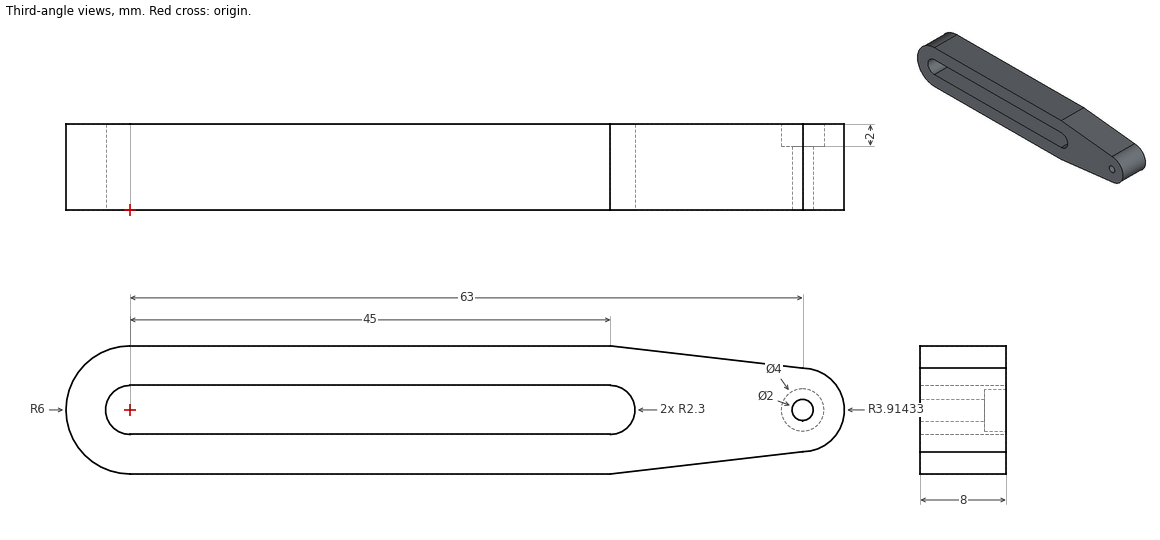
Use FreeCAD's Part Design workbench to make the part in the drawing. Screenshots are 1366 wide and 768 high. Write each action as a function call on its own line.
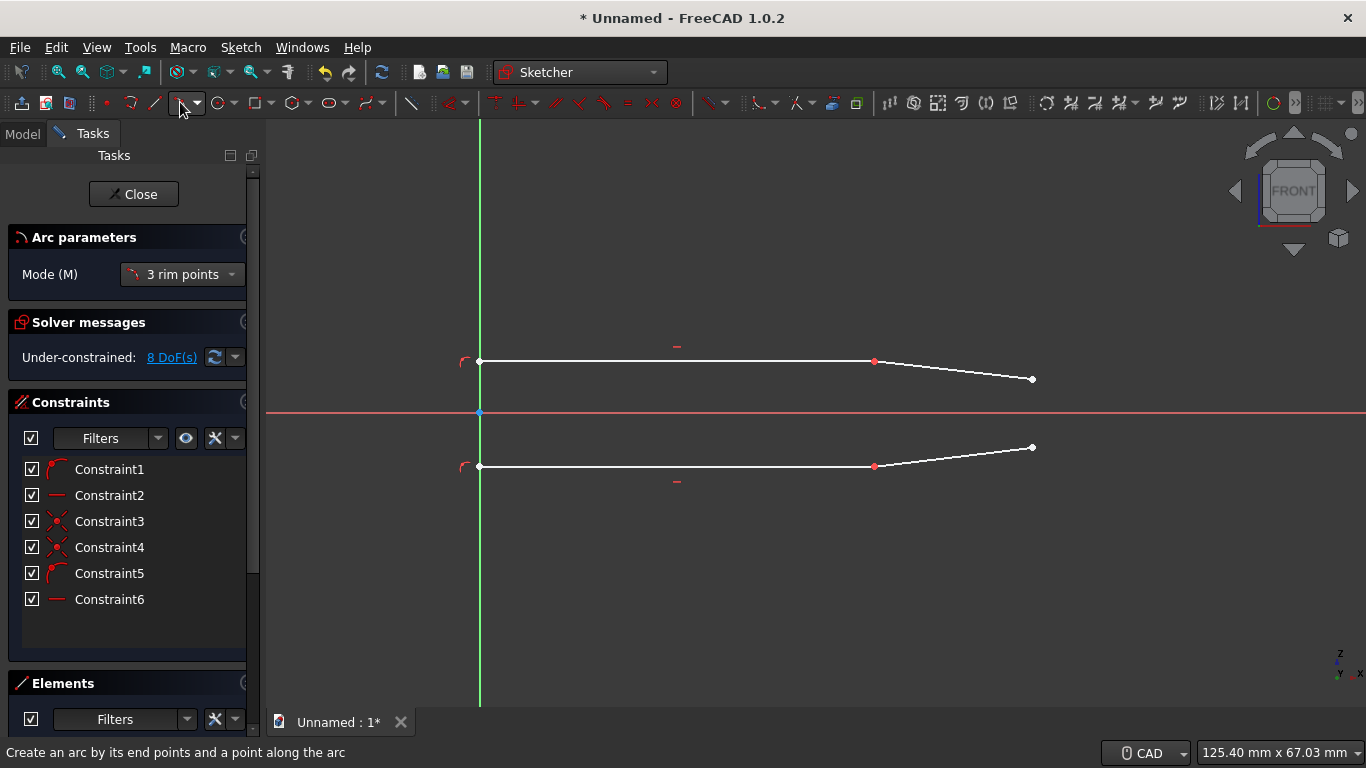
click(1032, 379)
click(1032, 448)
click(1060, 433)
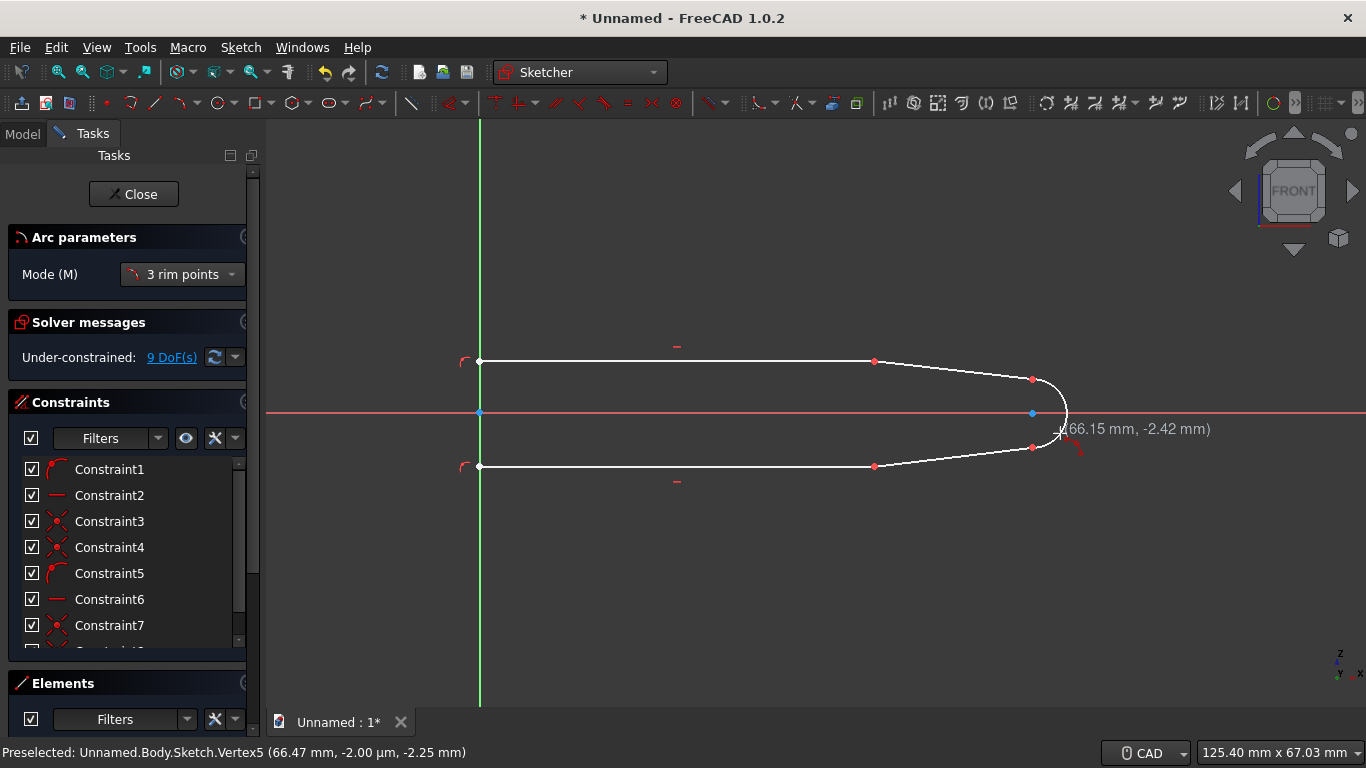
click(480, 467)
click(480, 361)
click(430, 396)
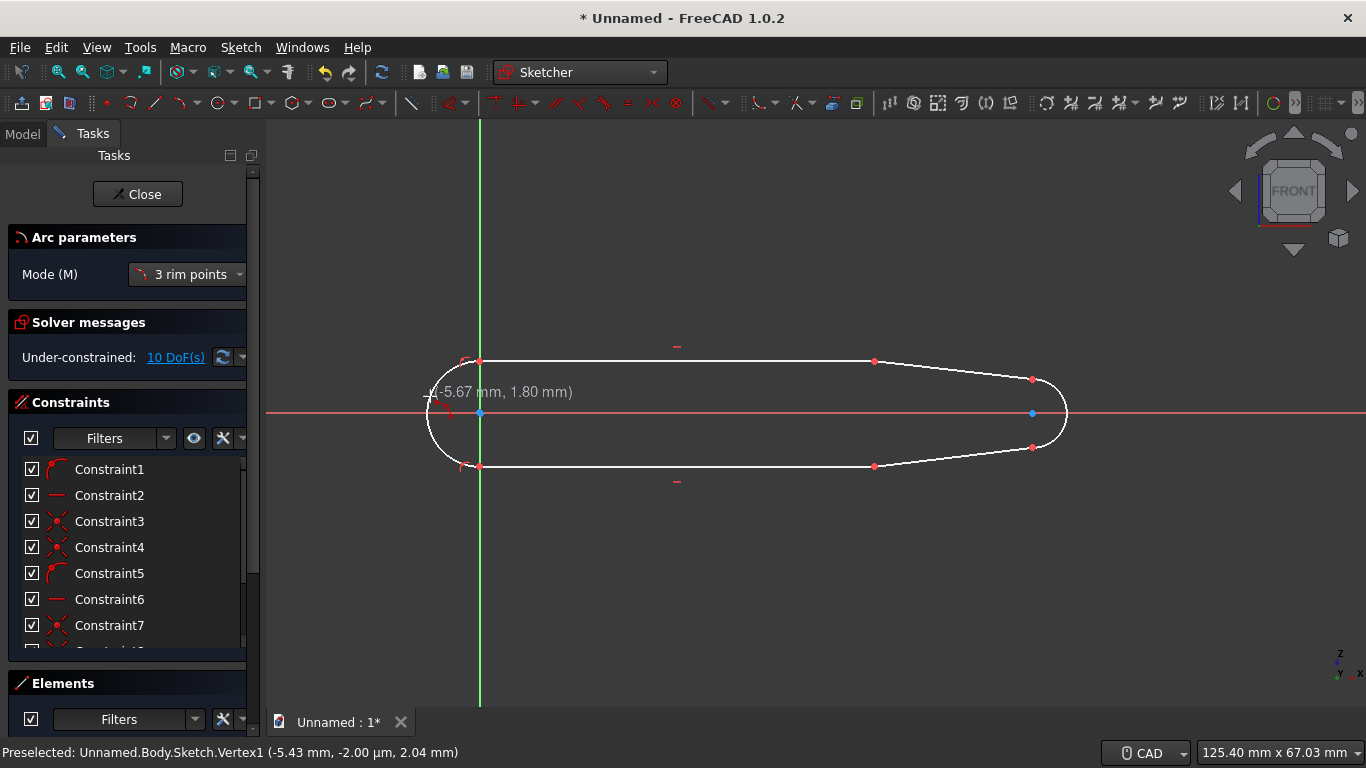
click(330, 104)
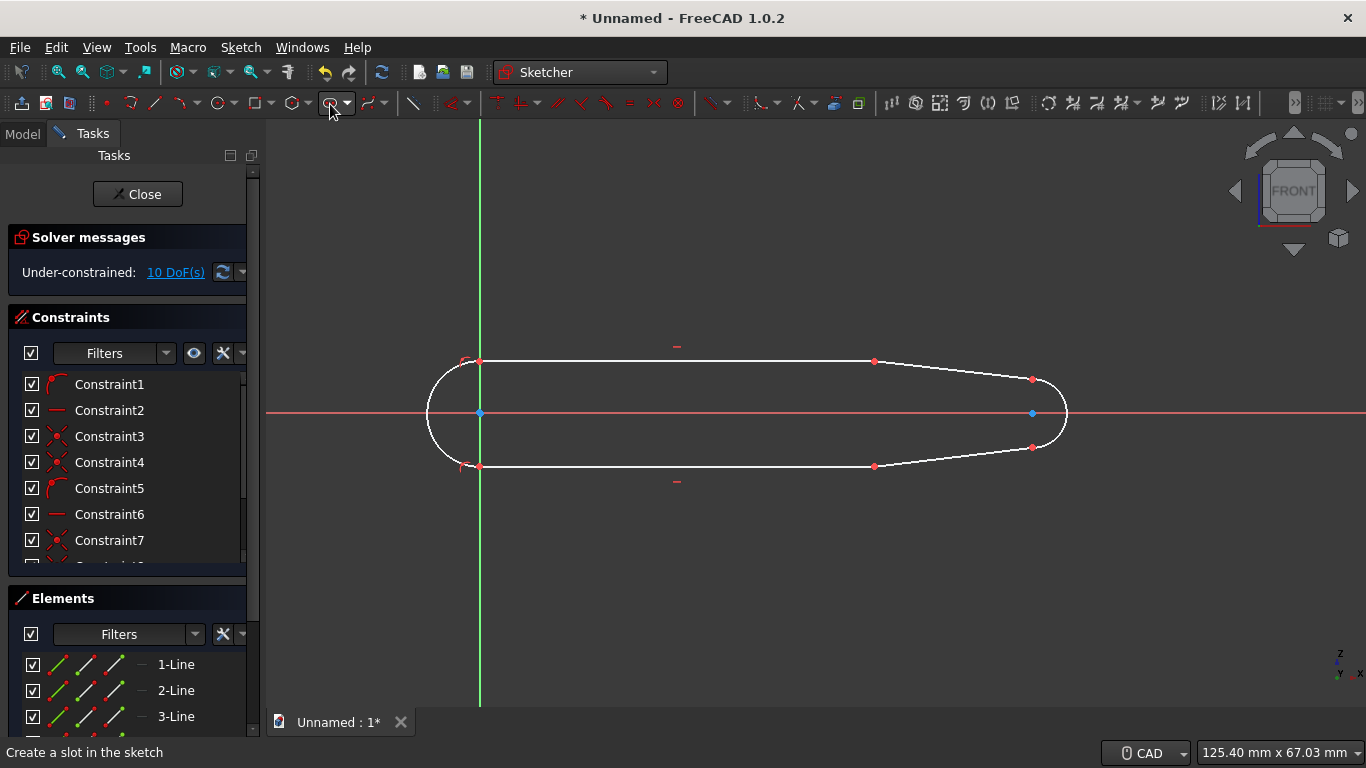
click(480, 413)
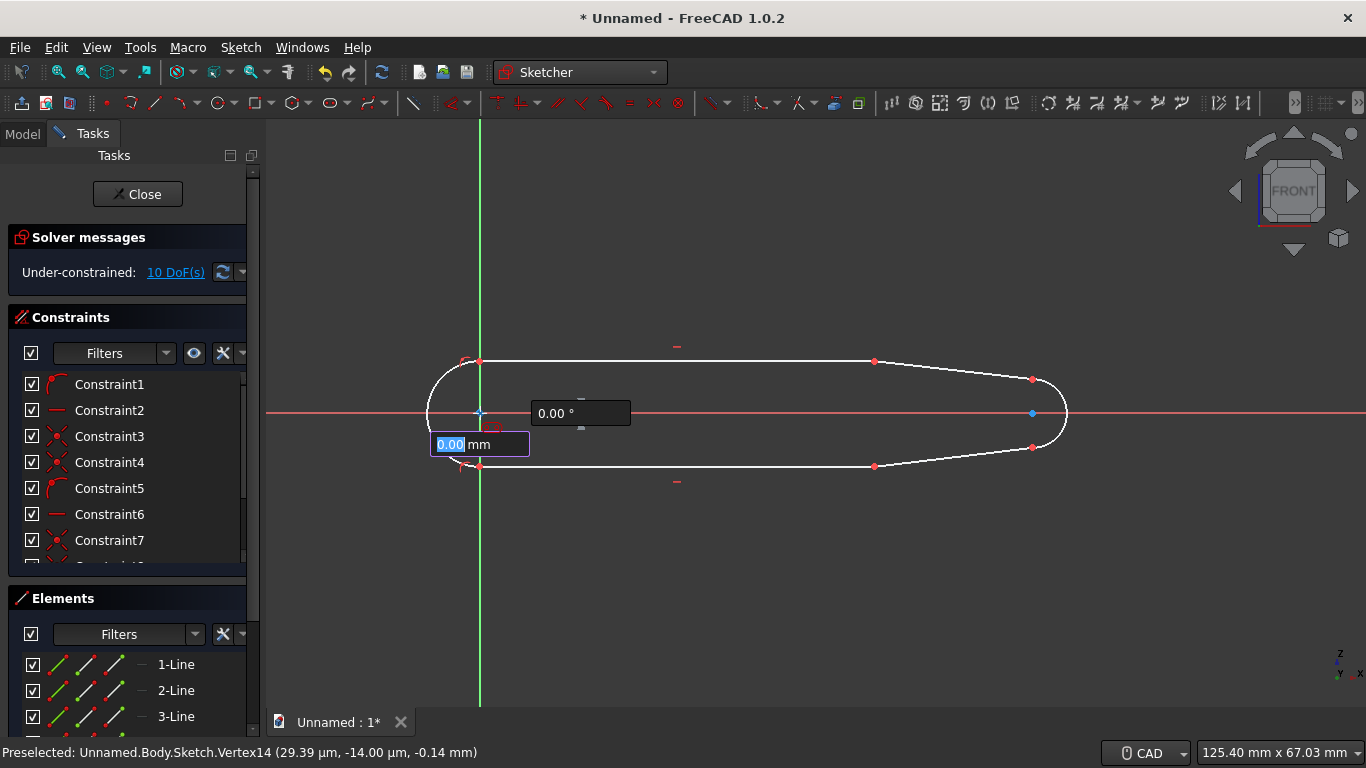
click(874, 404)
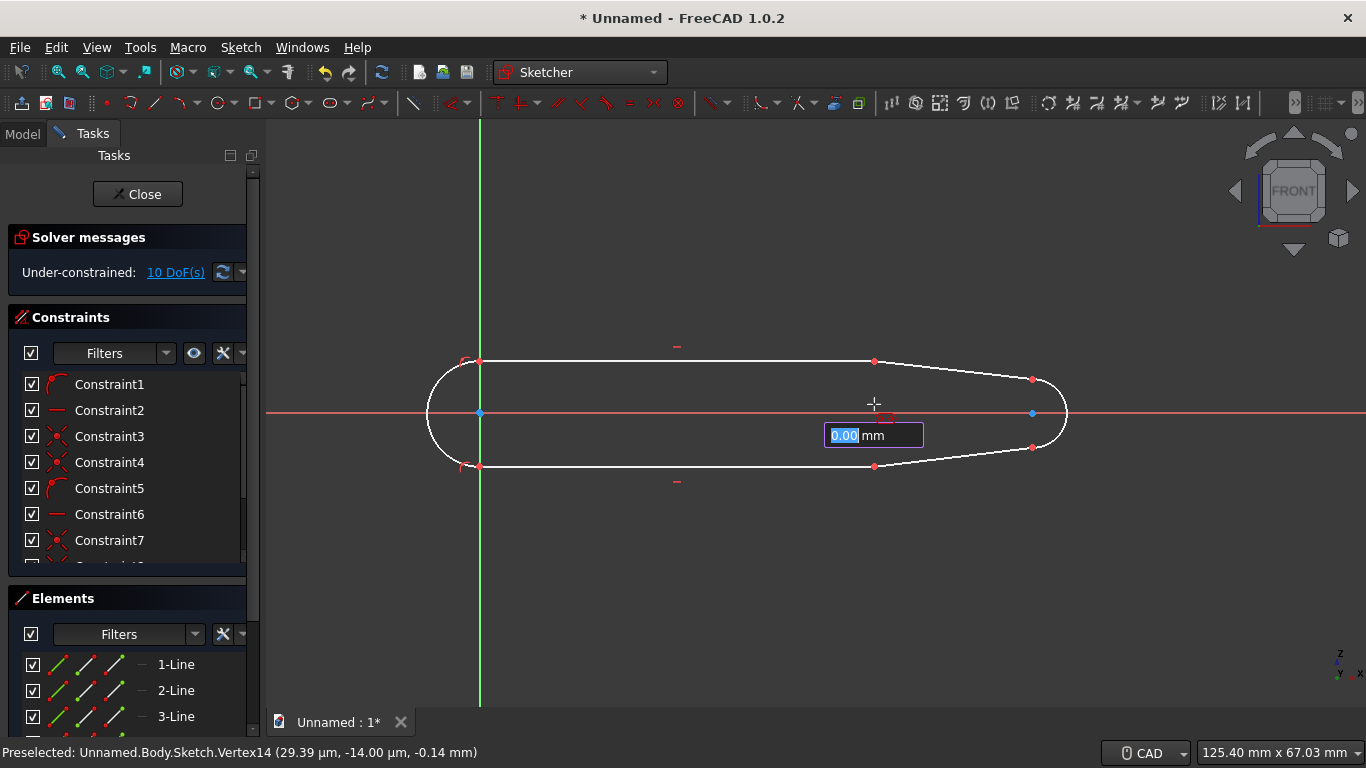
click(677, 433)
key(Escape)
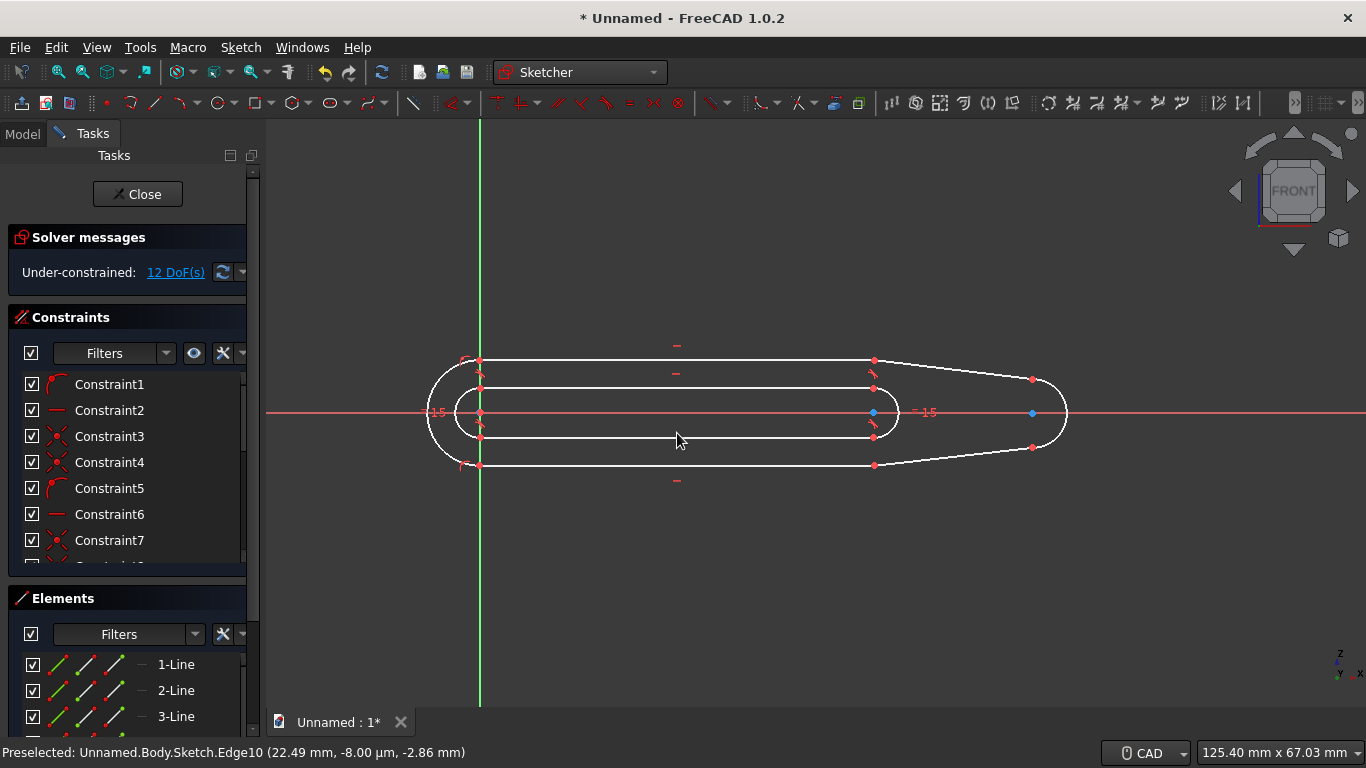
click(598, 360)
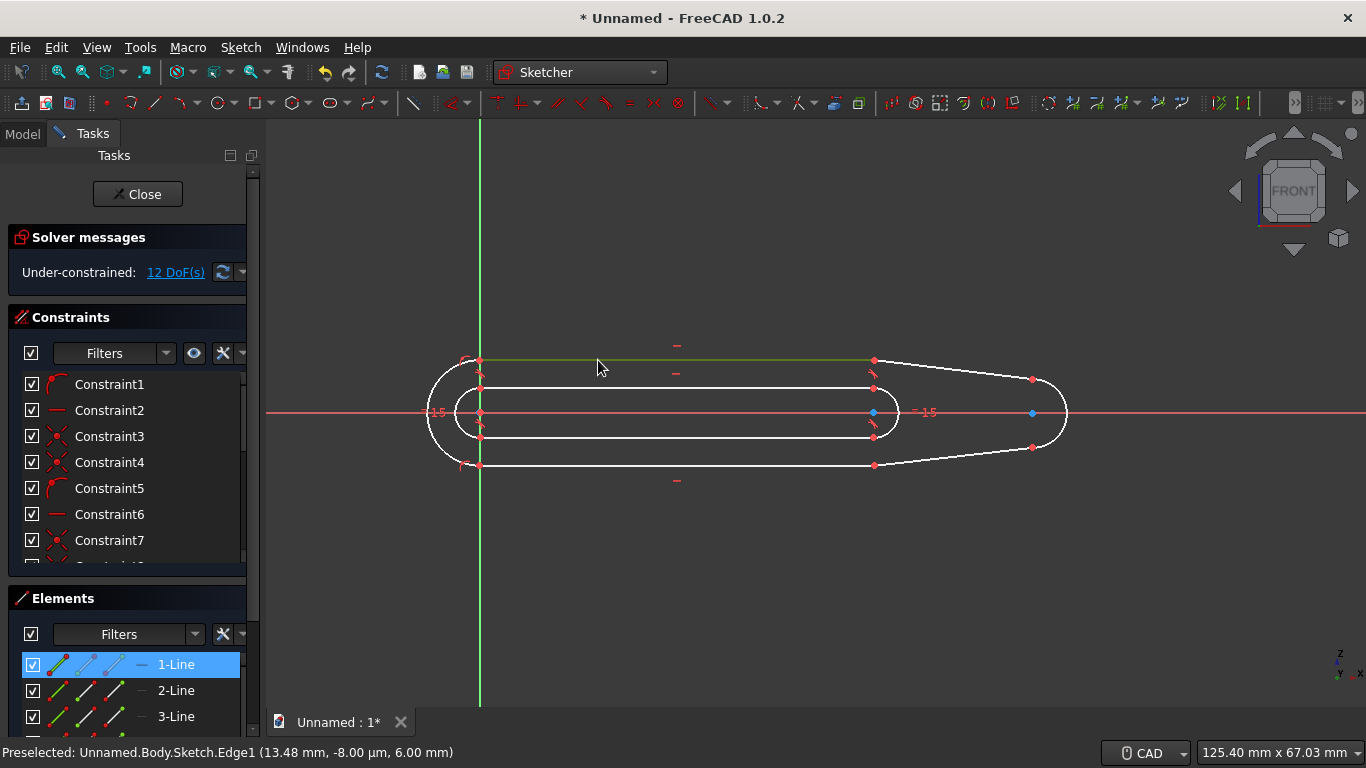
click(437, 382)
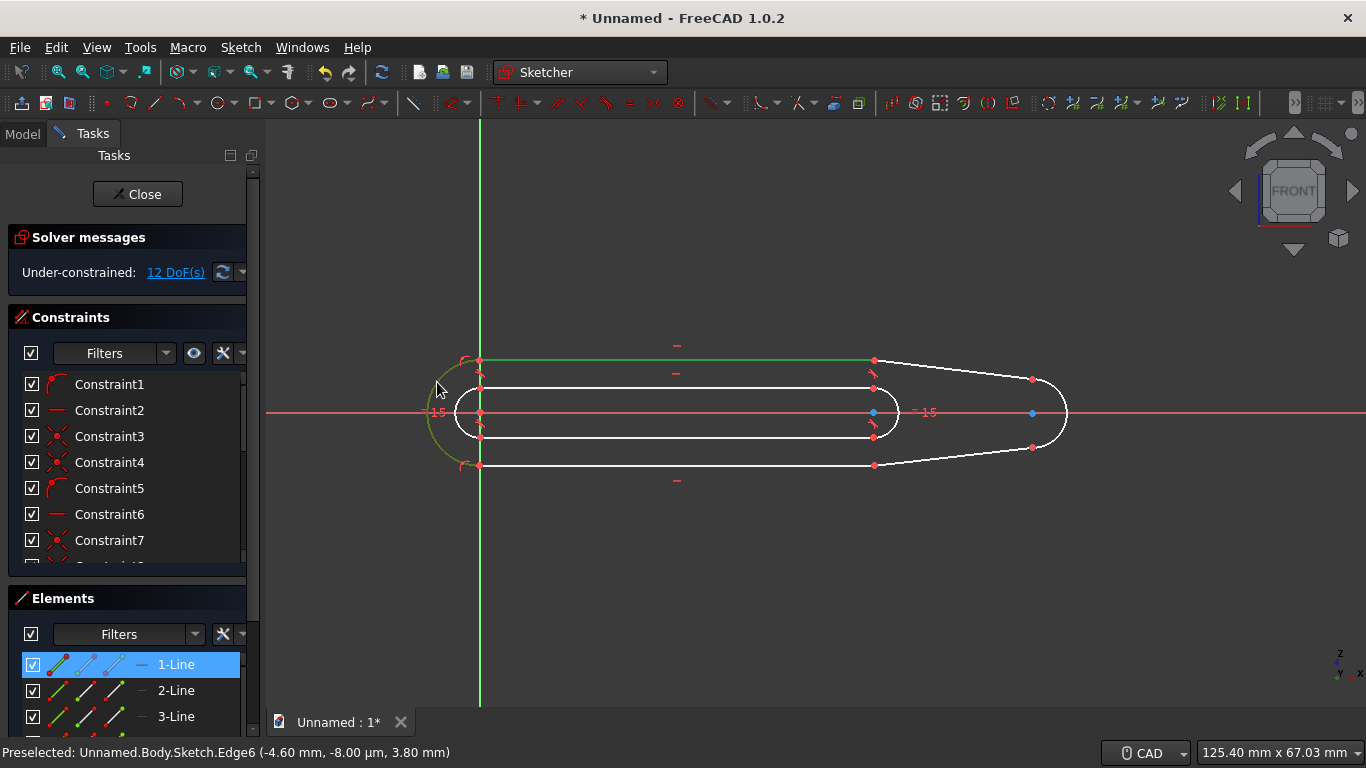
click(606, 104)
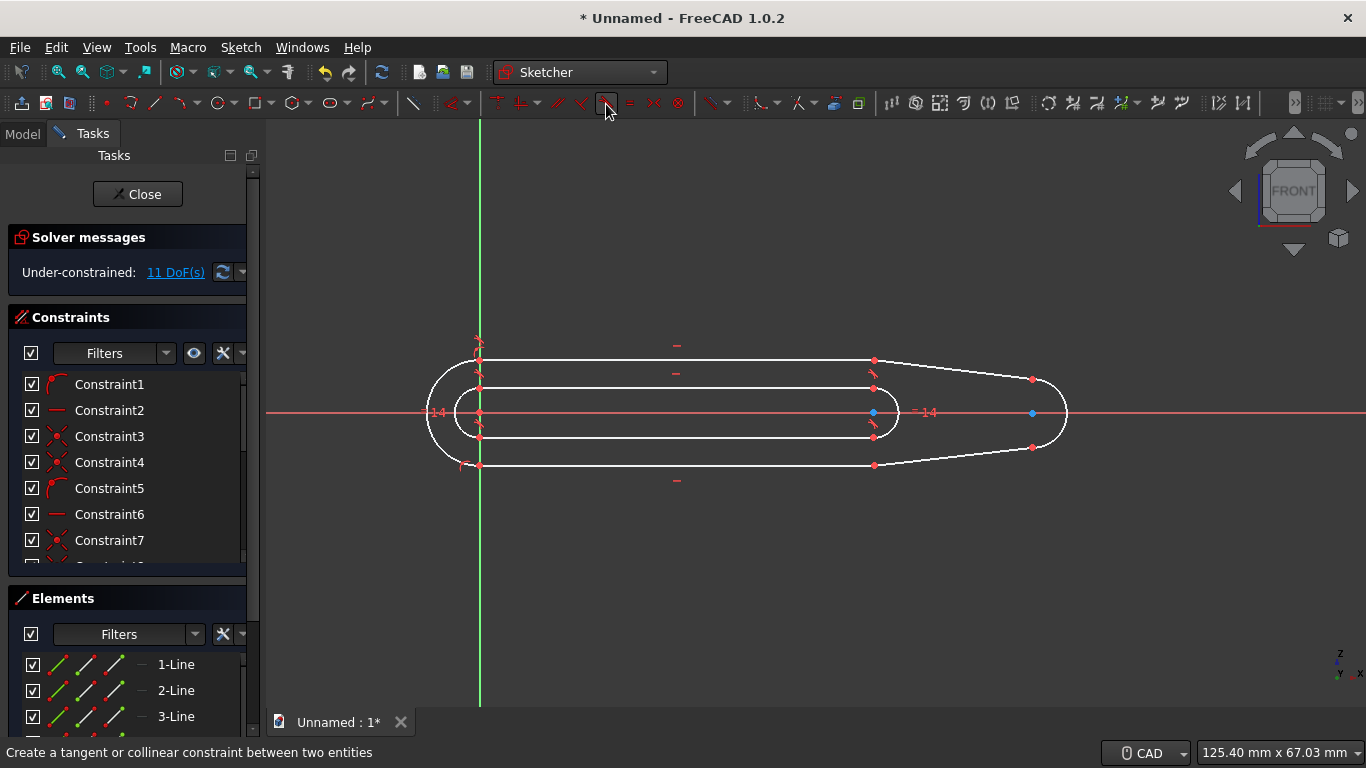
click(1032, 413)